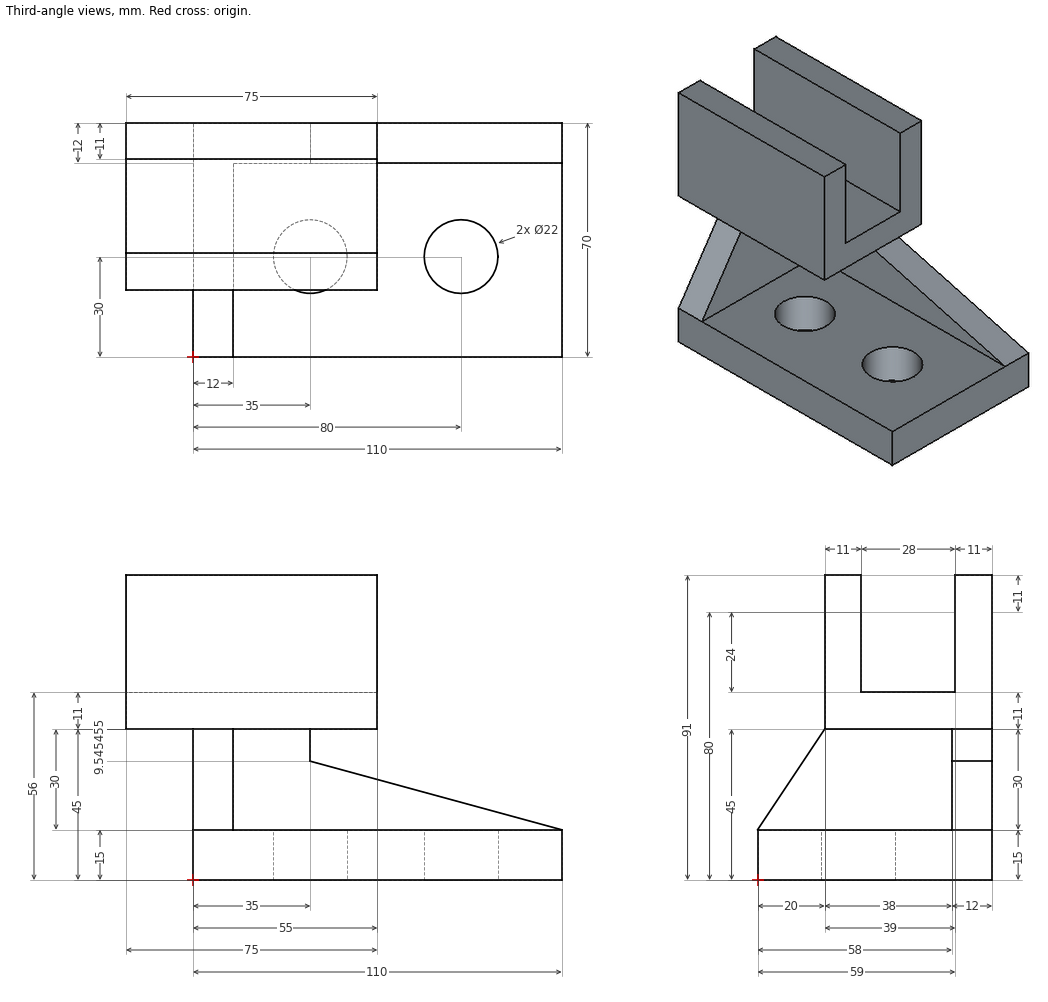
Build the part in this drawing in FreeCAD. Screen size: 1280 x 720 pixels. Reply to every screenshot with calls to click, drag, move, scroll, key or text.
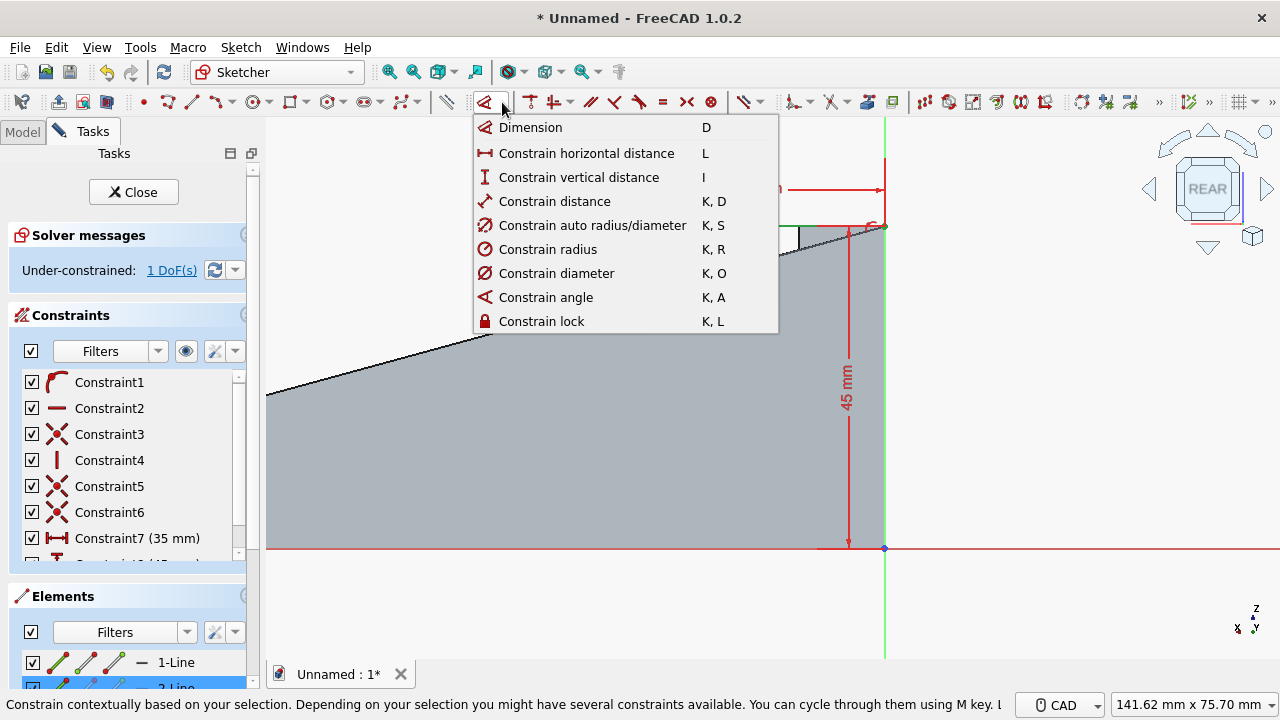
click(626, 177)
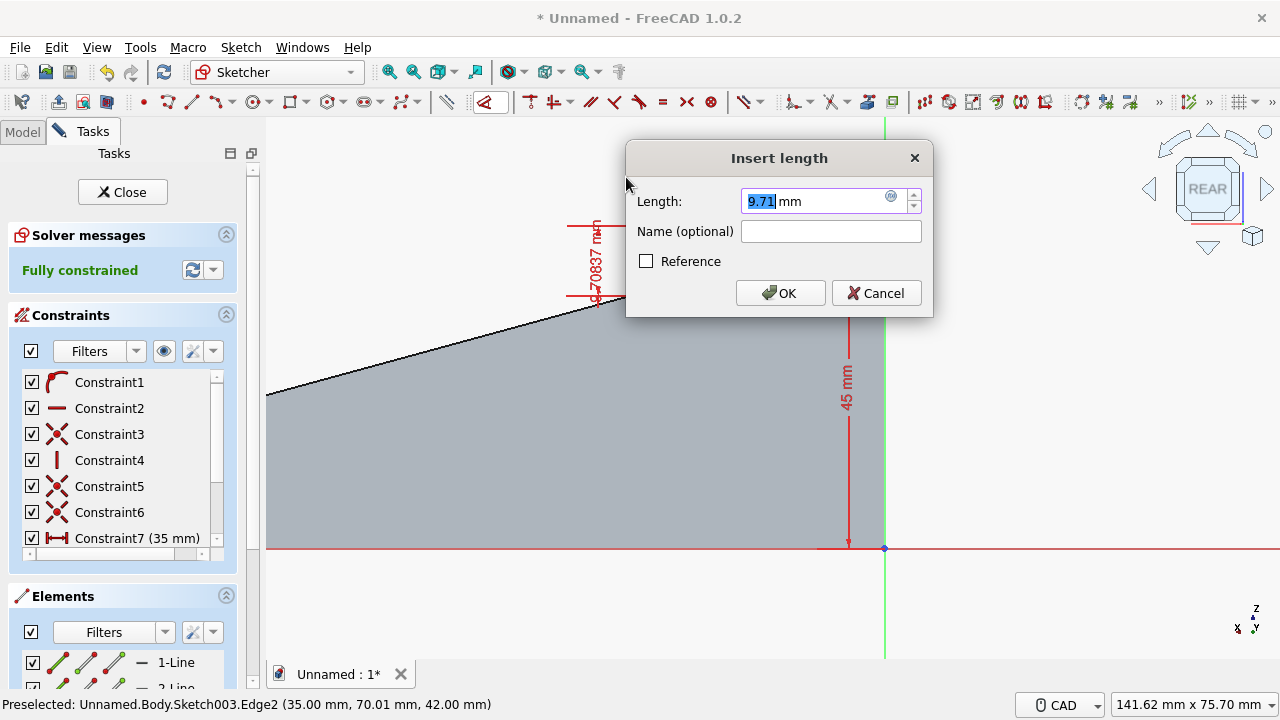
text(9.545455)
key(Return)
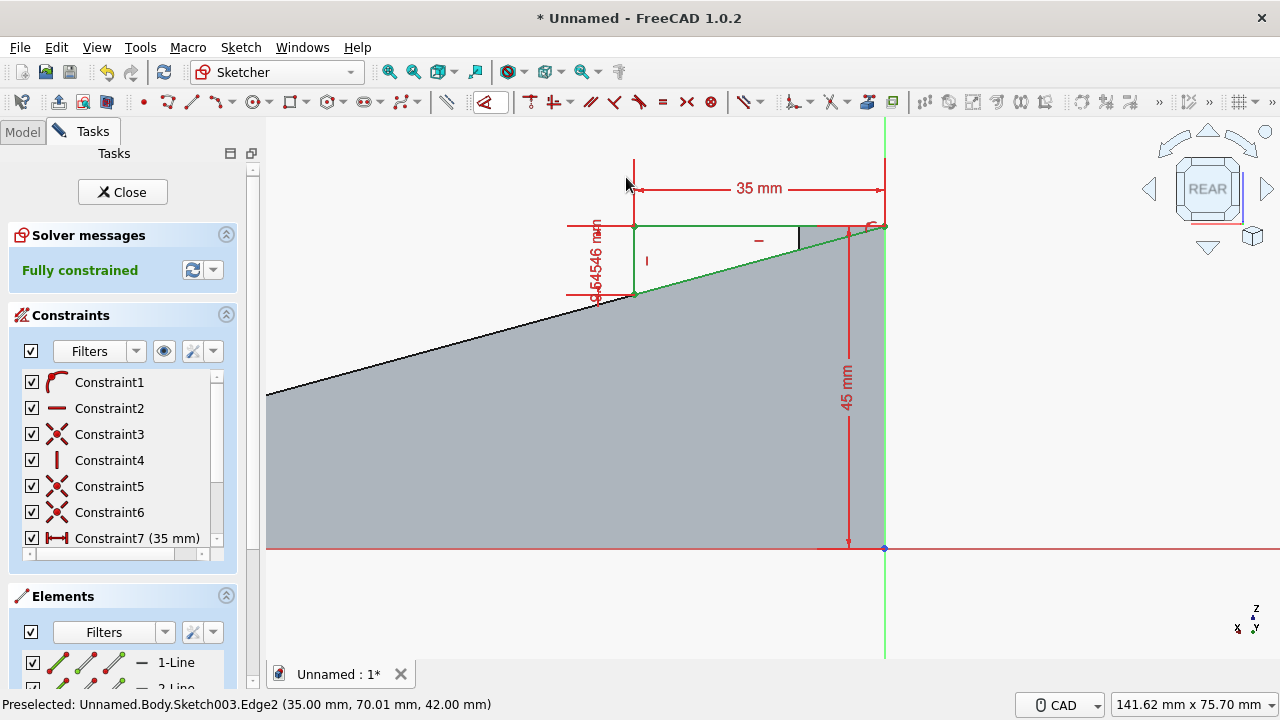
click(123, 192)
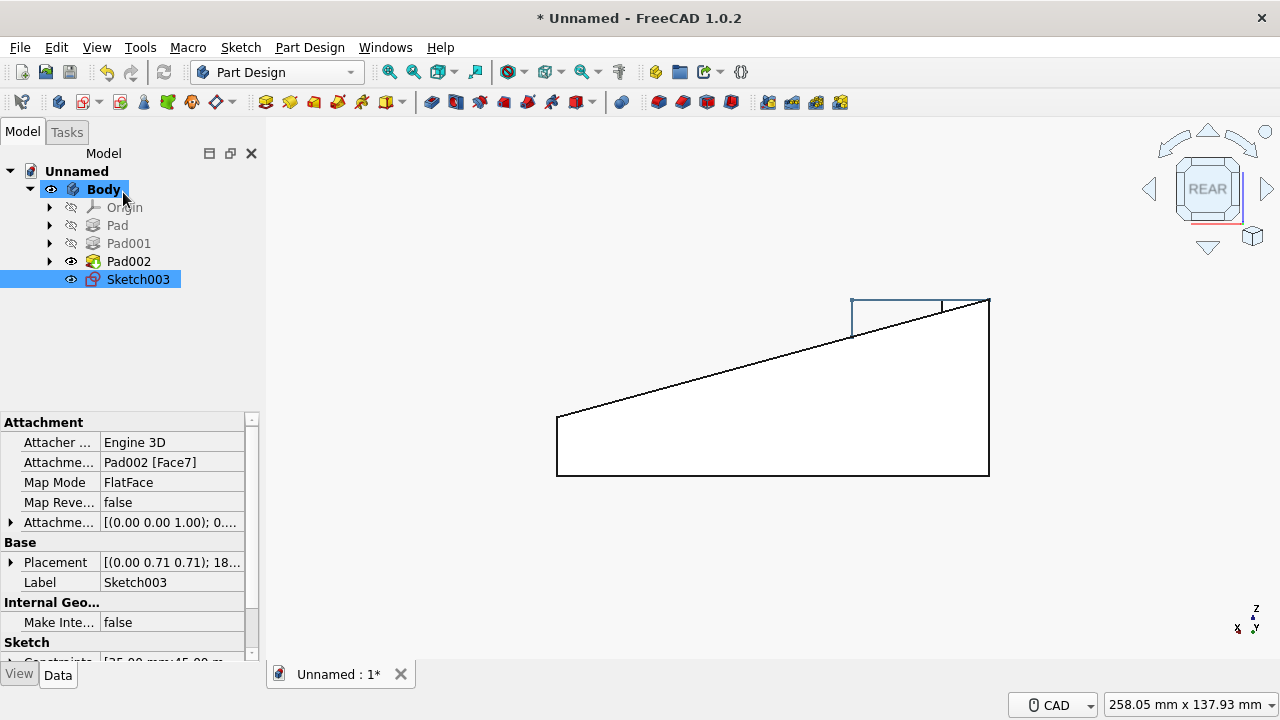
click(266, 102)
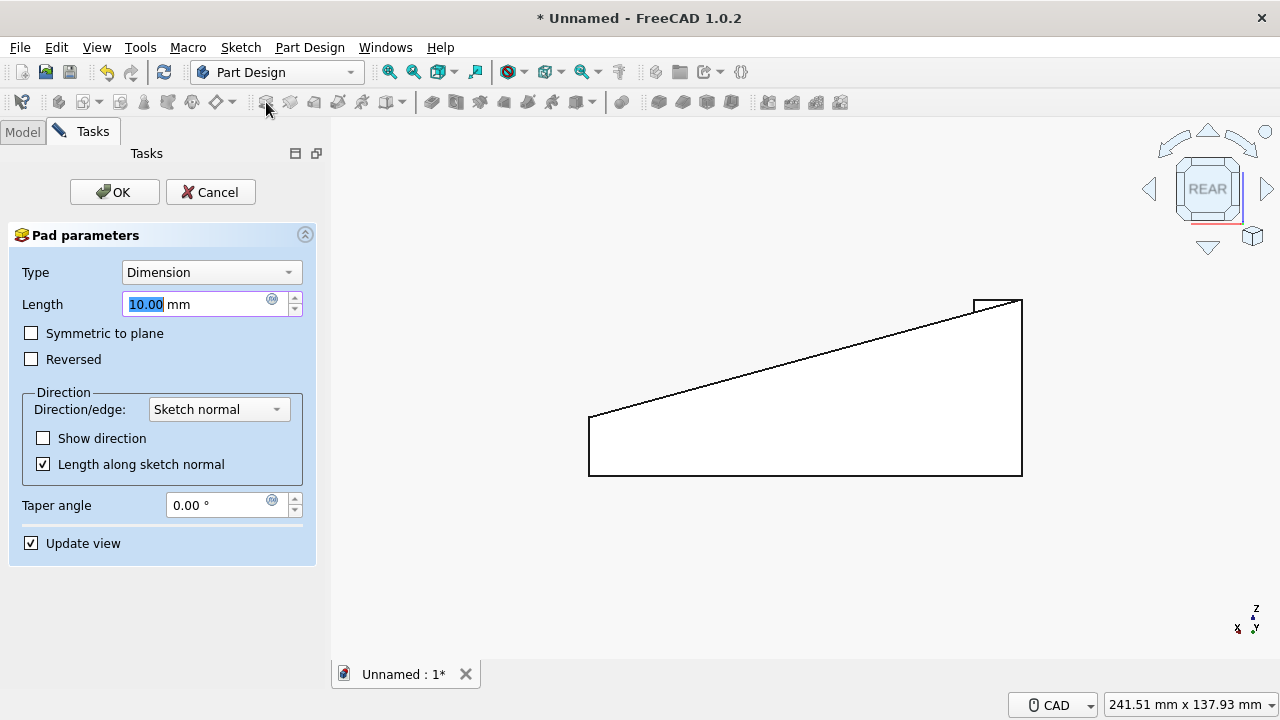
text(12)
key(Tab)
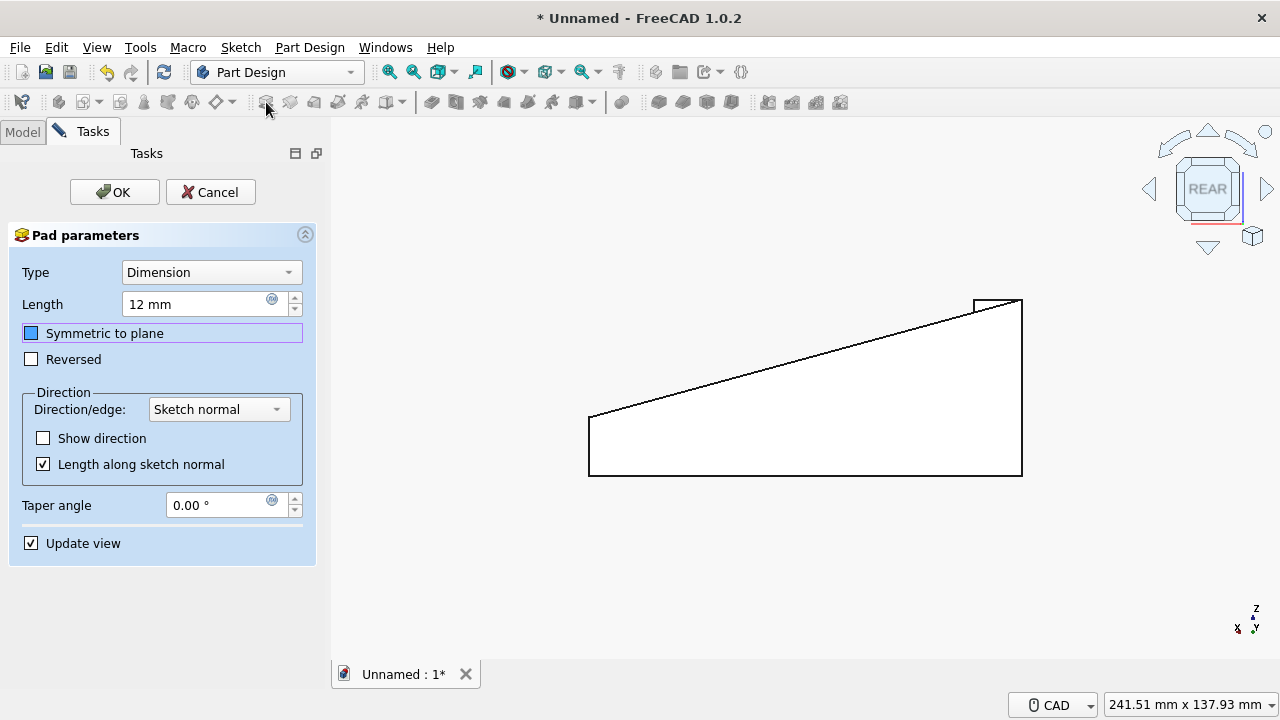
click(30, 359)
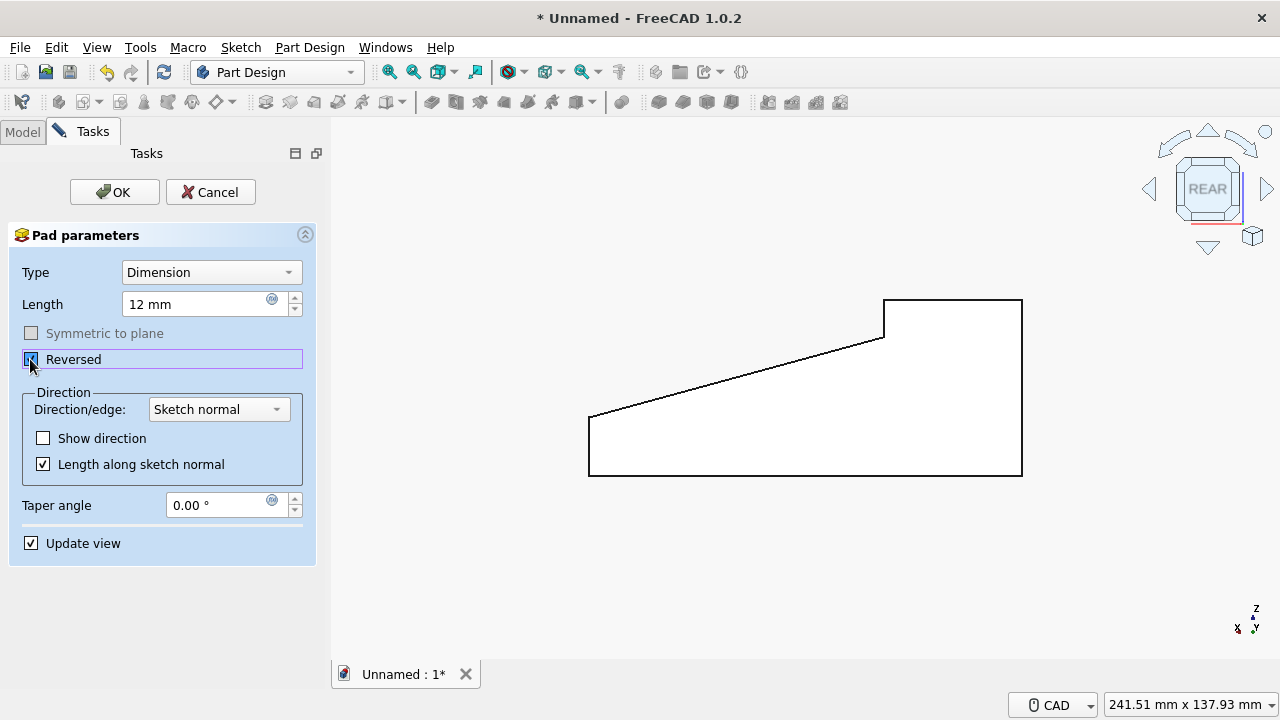
click(115, 192)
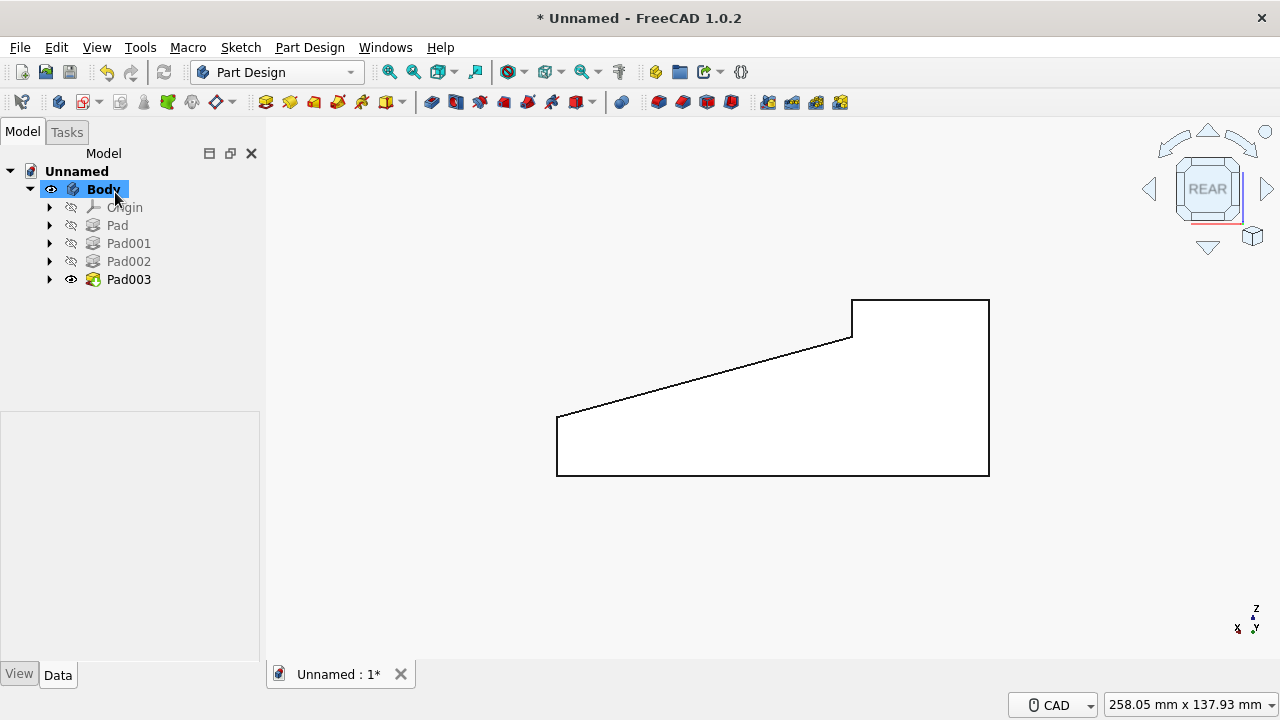
click(390, 72)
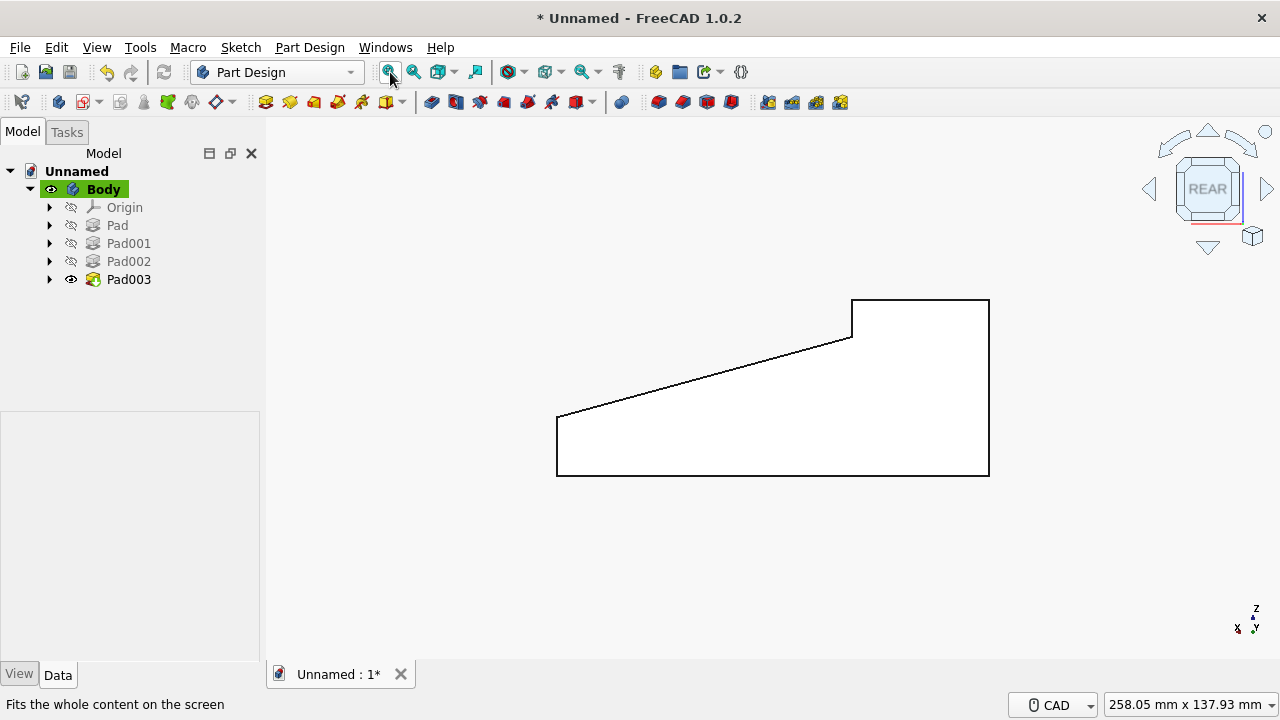
click(896, 387)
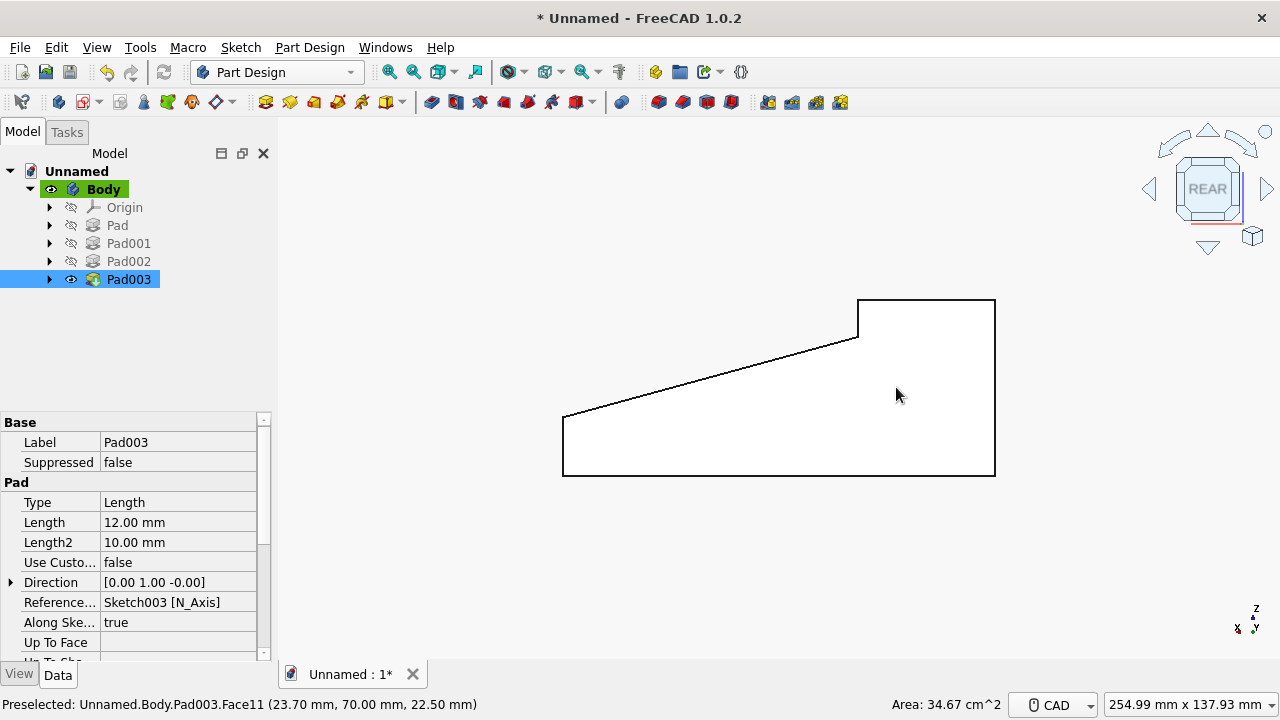
click(84, 102)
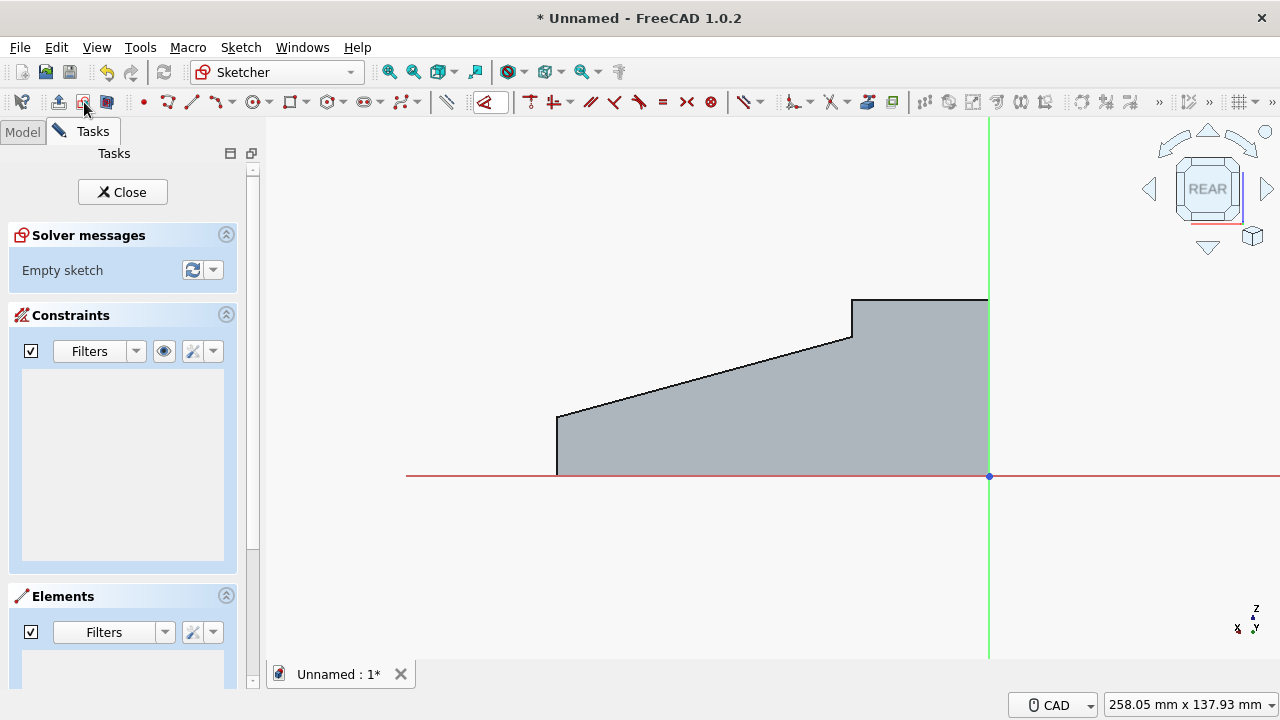
scroll(1115, 322, up, 2)